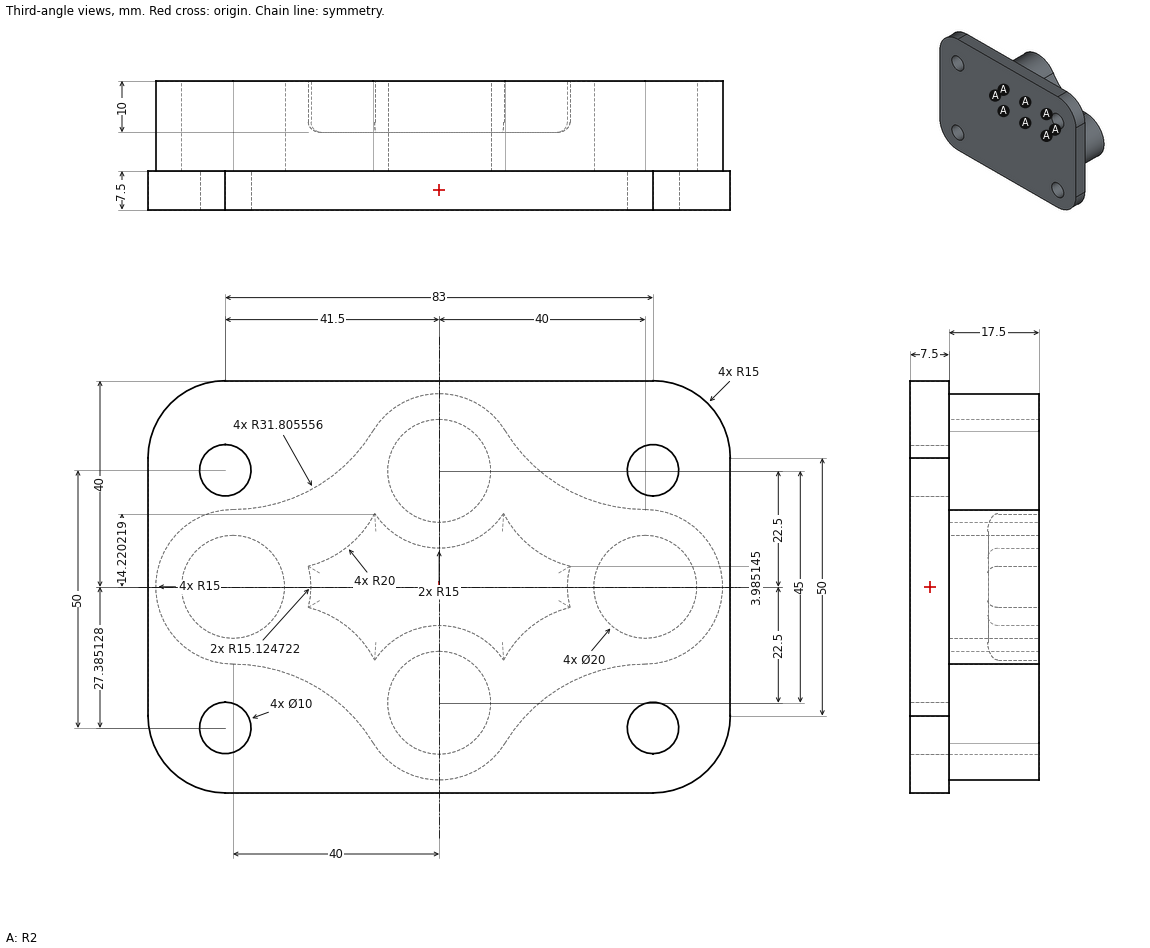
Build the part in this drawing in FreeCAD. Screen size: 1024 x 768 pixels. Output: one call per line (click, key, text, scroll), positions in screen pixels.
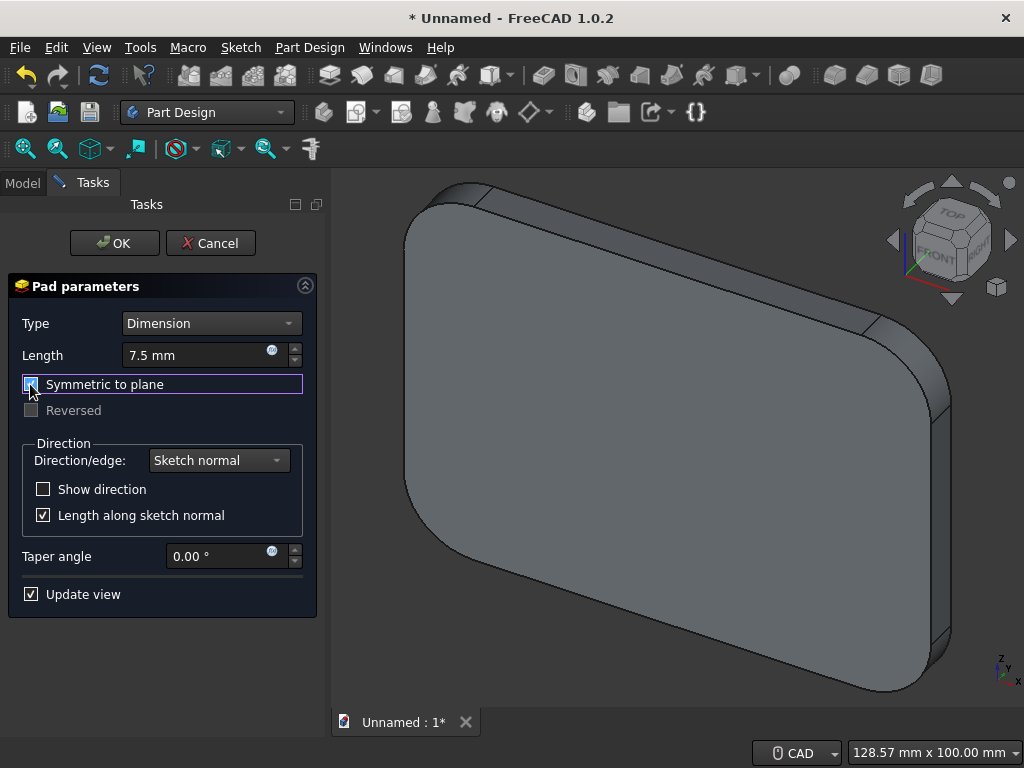
click(115, 243)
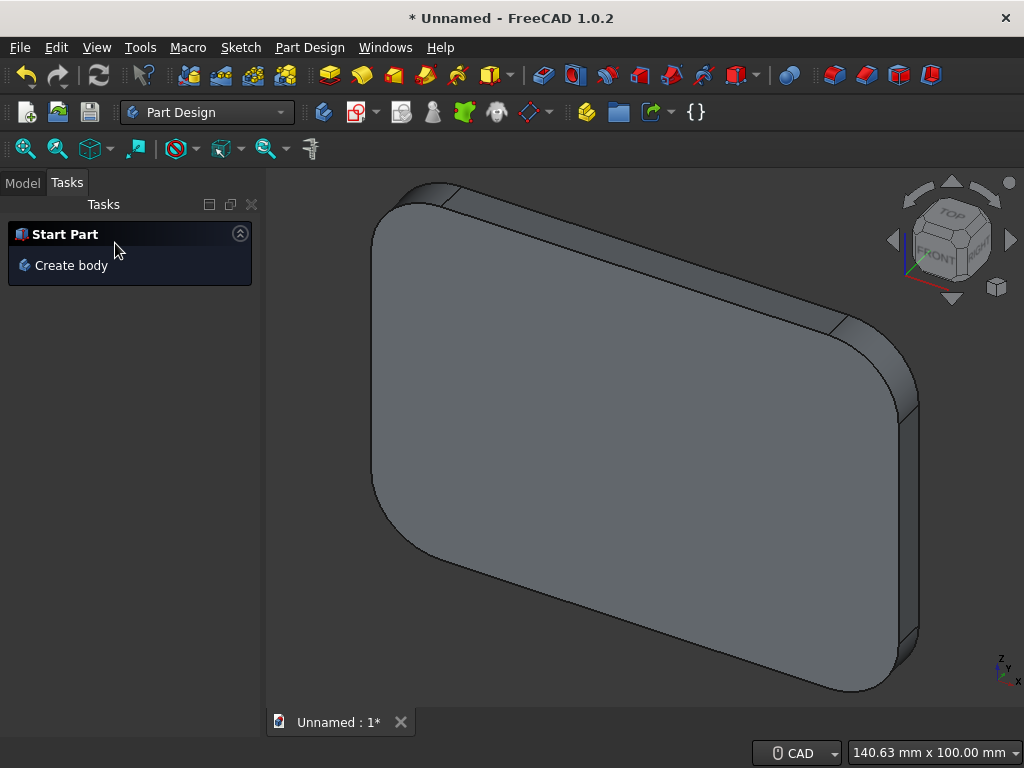
click(26, 150)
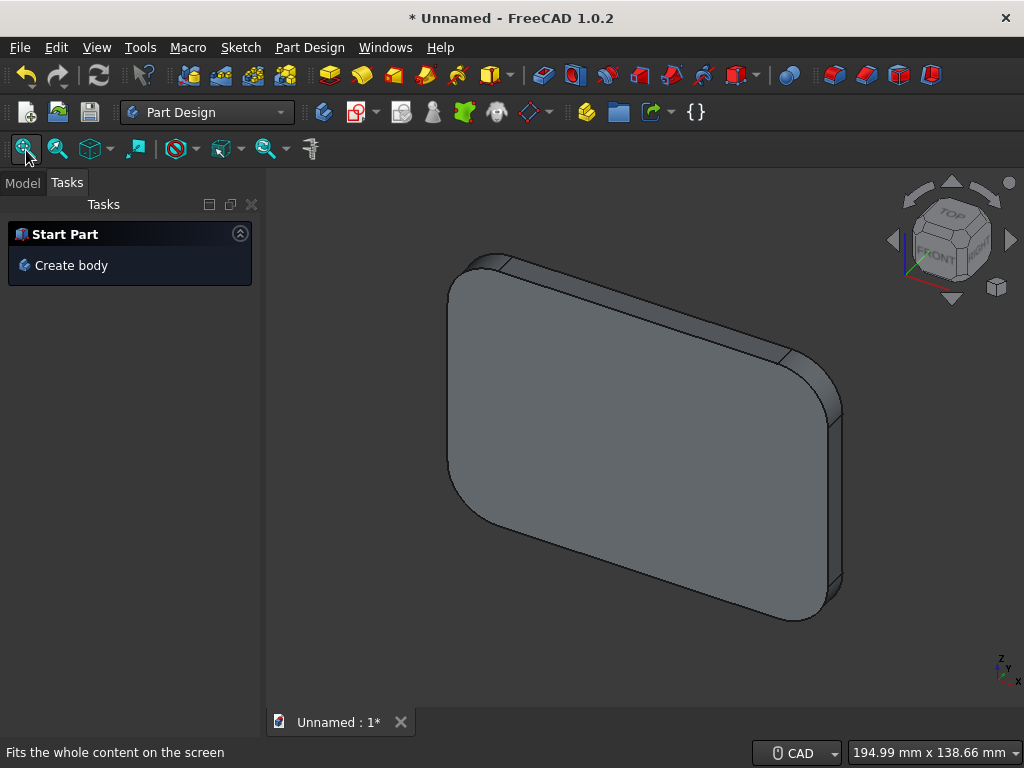
key(4)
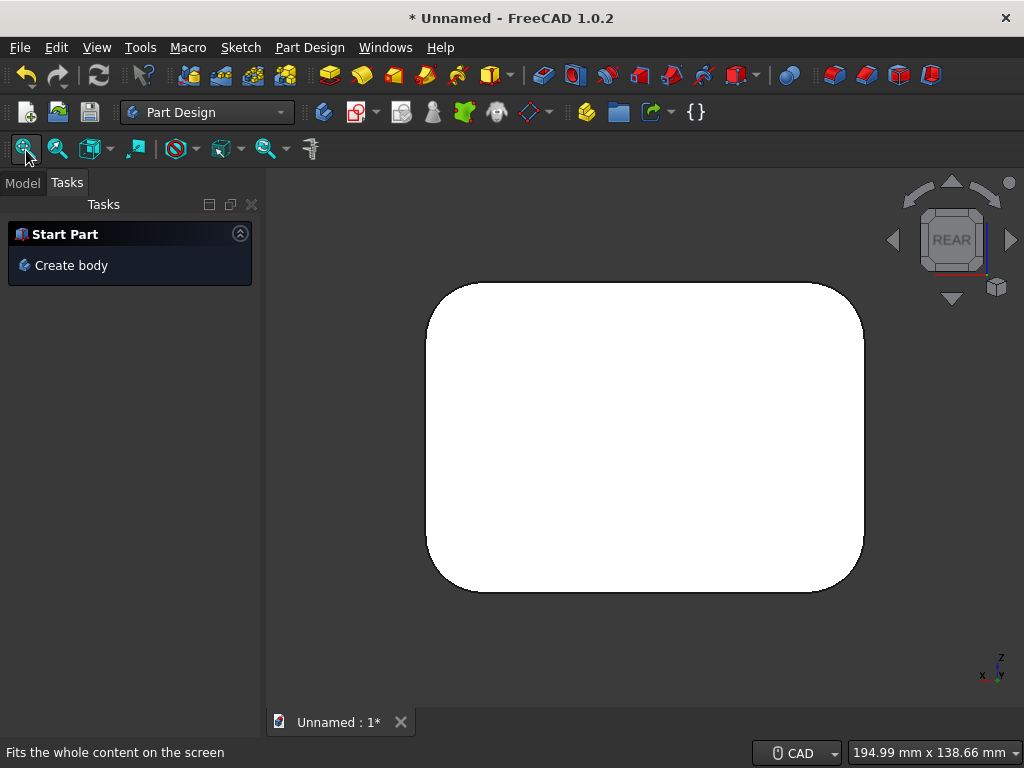
click(582, 436)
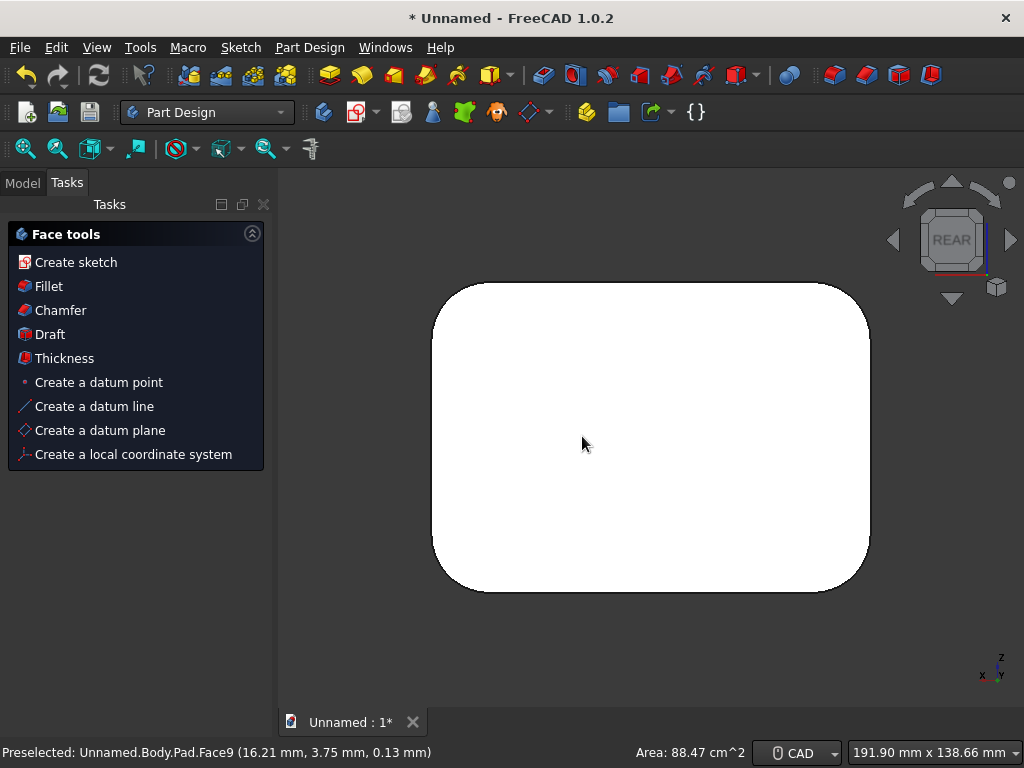
click(356, 112)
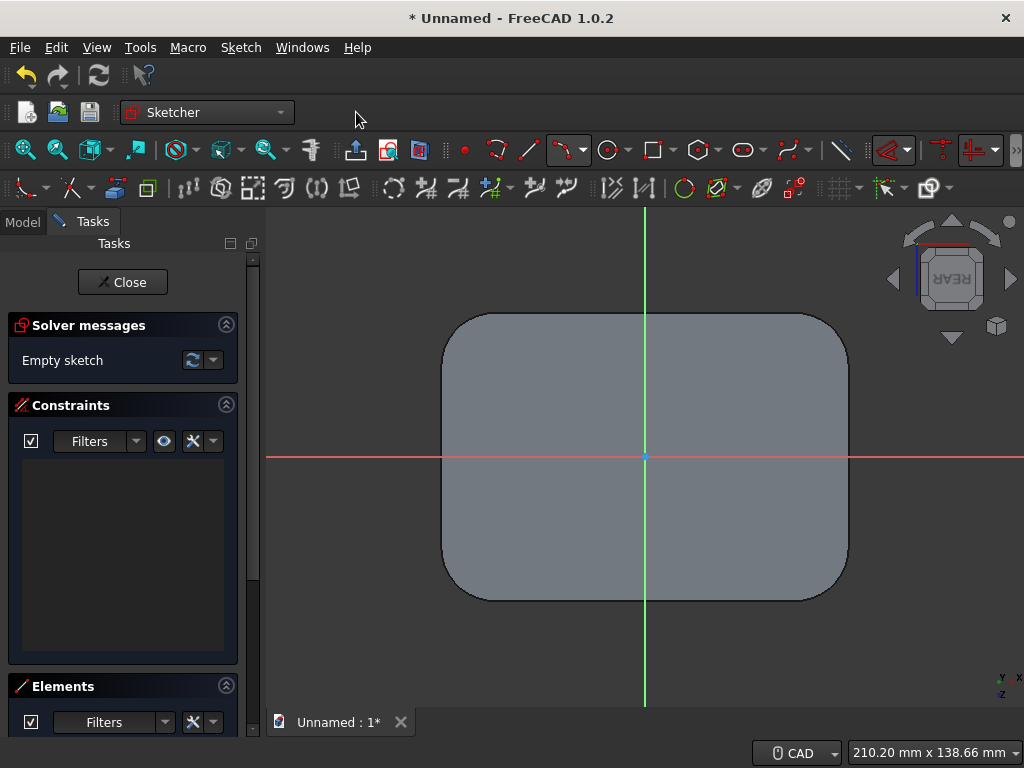
click(608, 150)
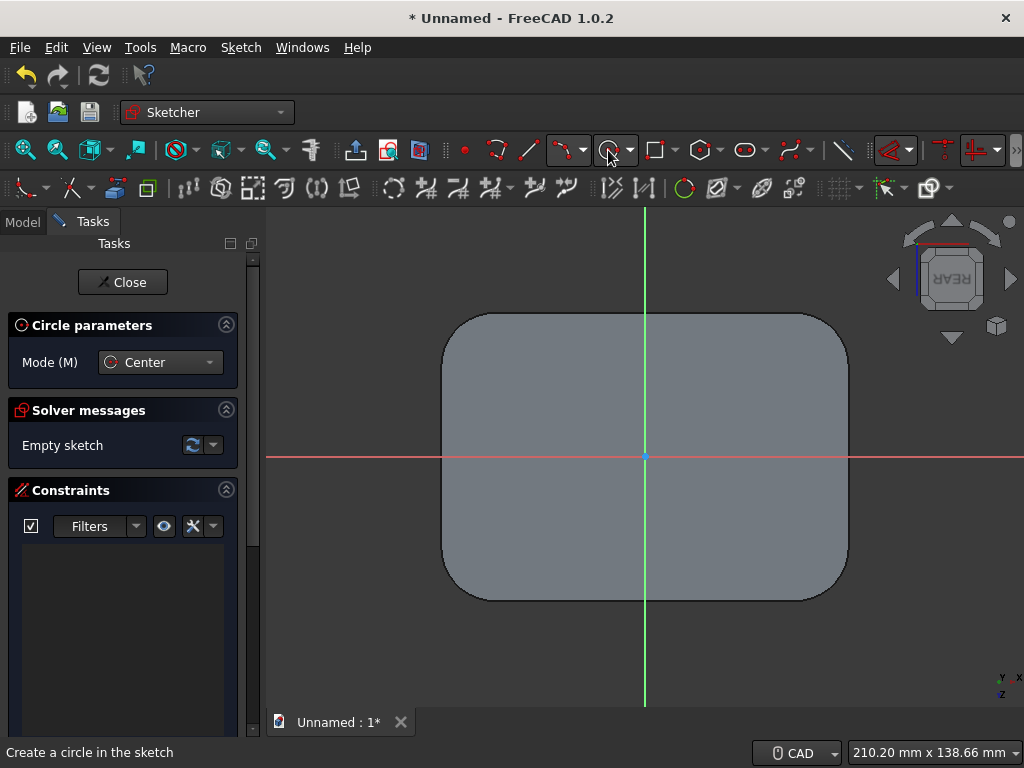
scroll(495, 358, up, 2)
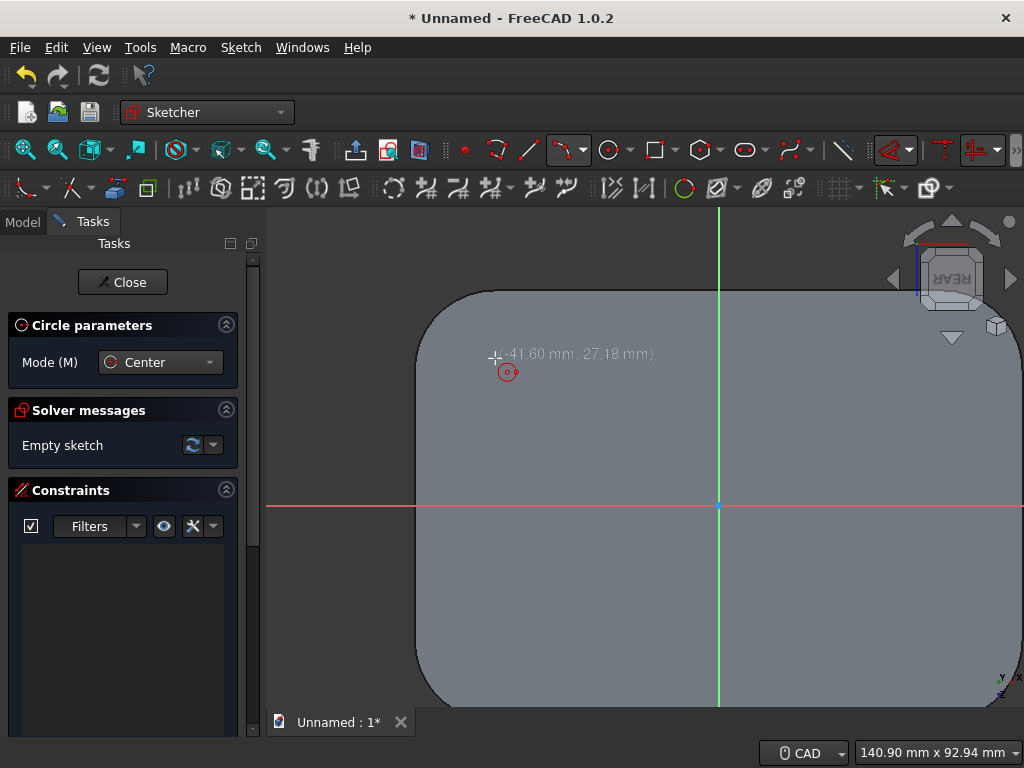
click(495, 358)
move(514, 339)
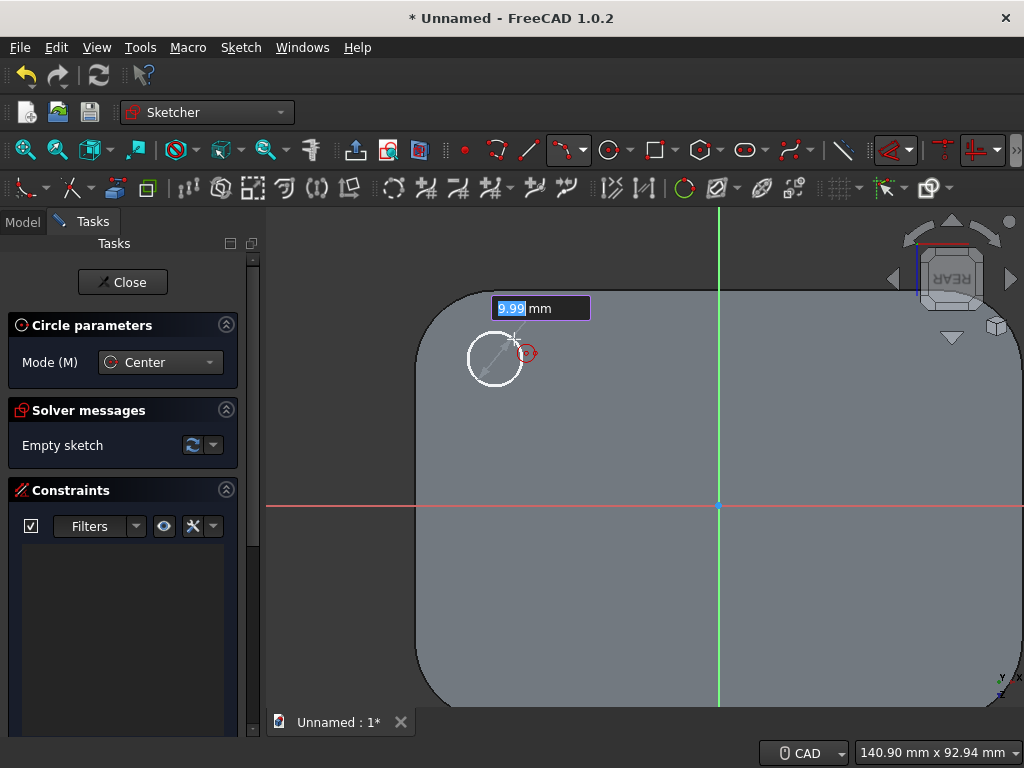
text(10)
key(Return)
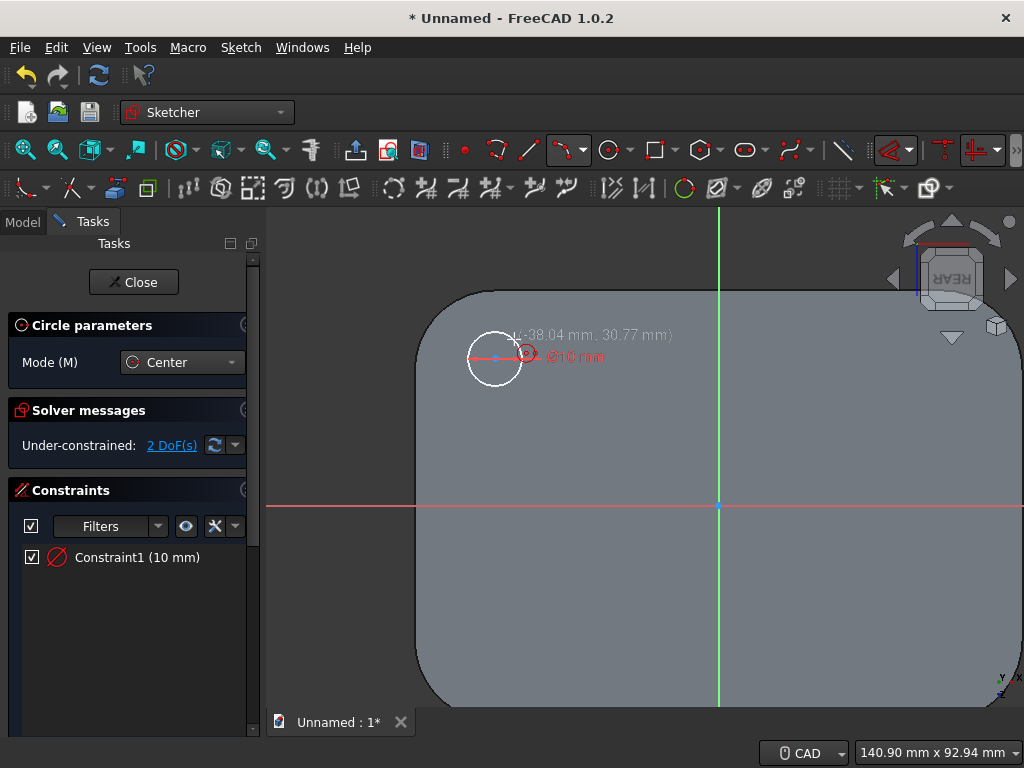
click(495, 627)
move(514, 608)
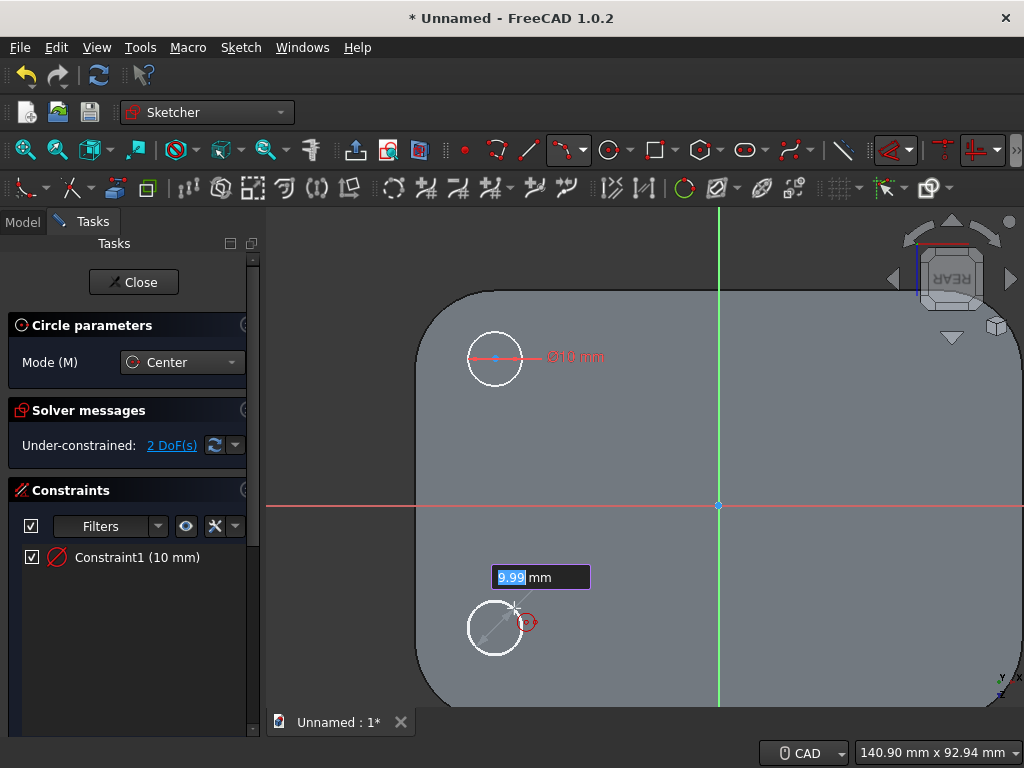
text(10)
key(Return)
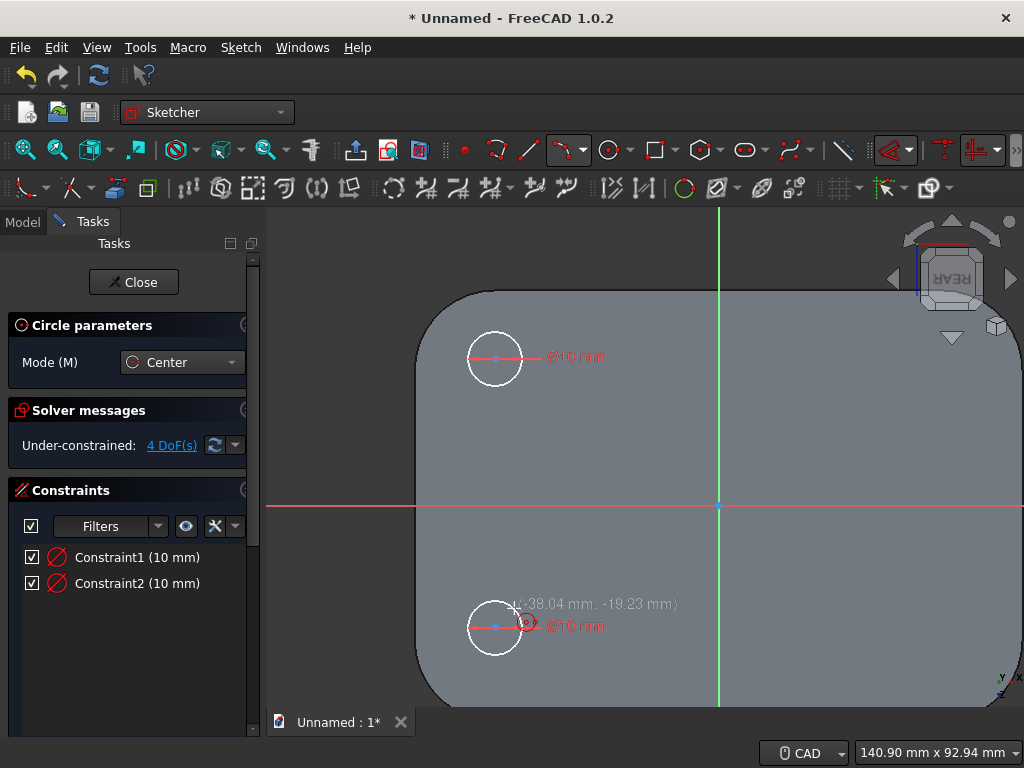
scroll(294, 384, down, 2)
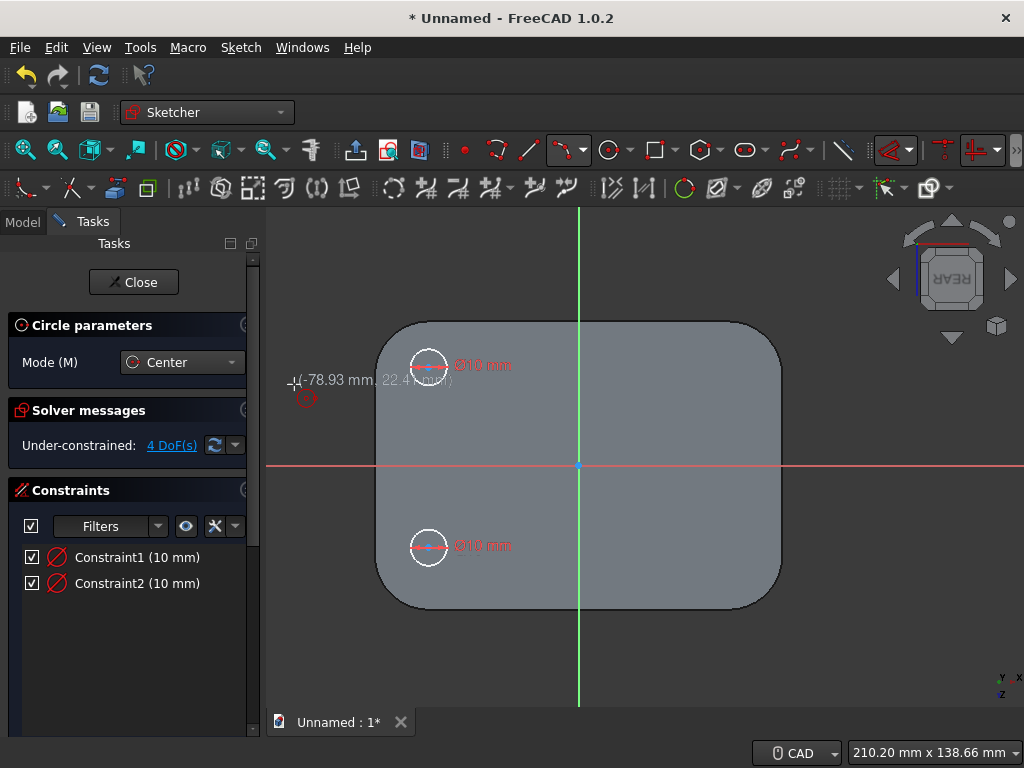
scroll(728, 547, up, 2)